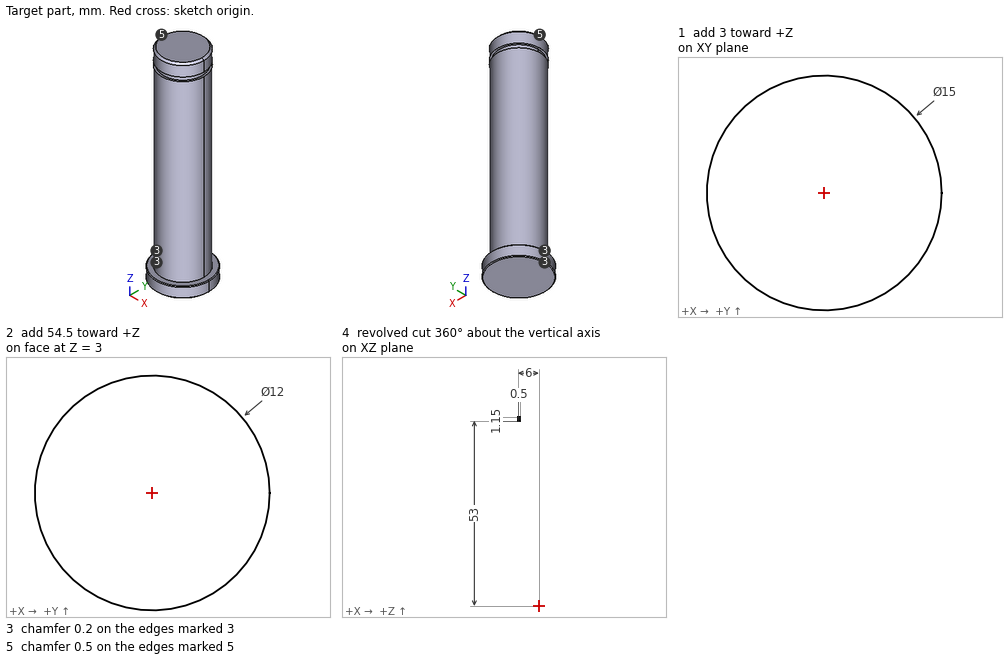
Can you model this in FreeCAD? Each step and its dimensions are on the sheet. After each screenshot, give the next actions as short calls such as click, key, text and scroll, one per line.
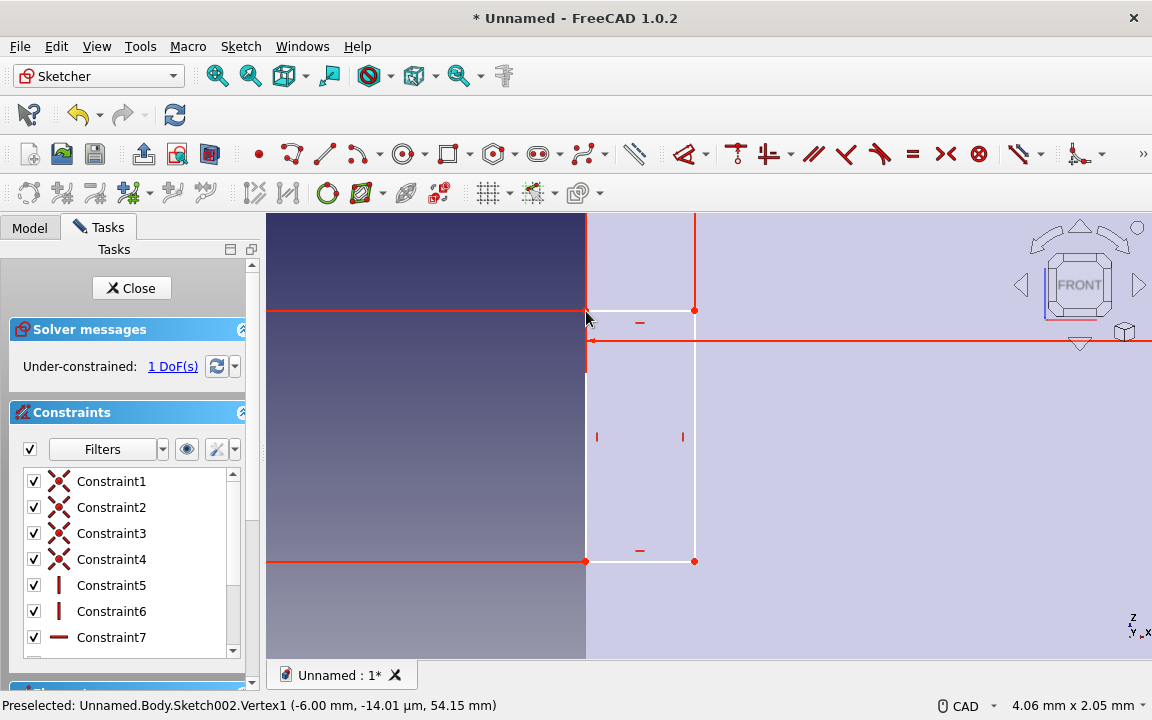
click(586, 562)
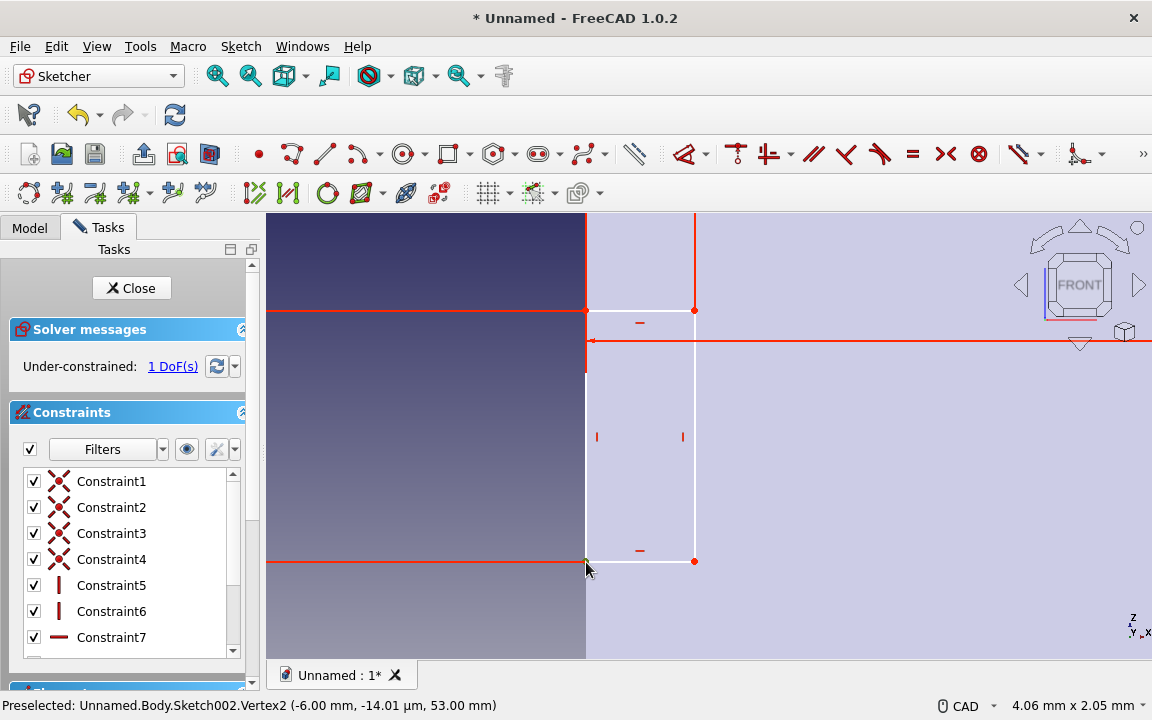
key(i)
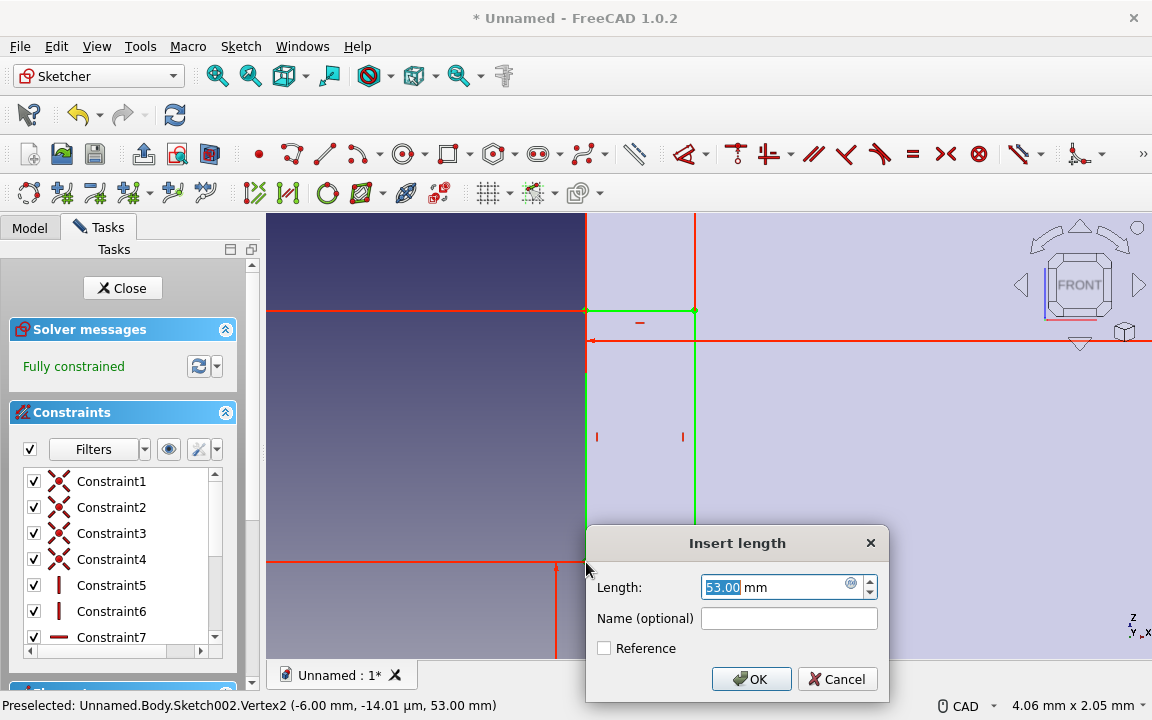
text(53)
key(Return)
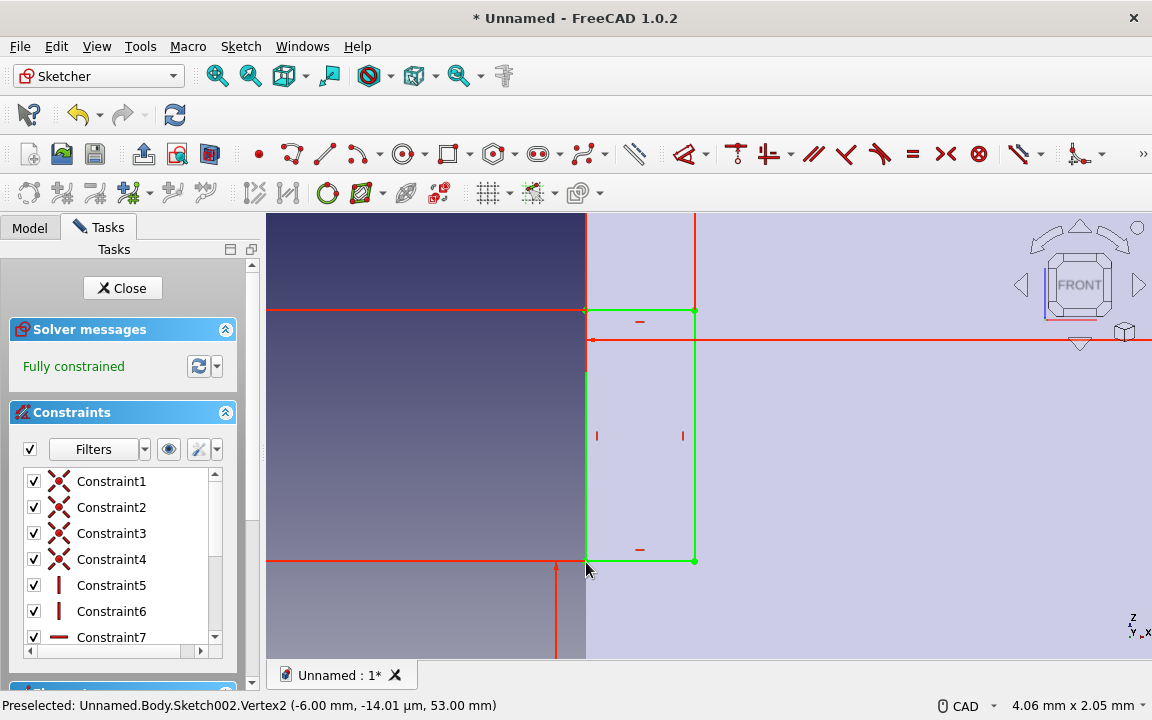
click(123, 288)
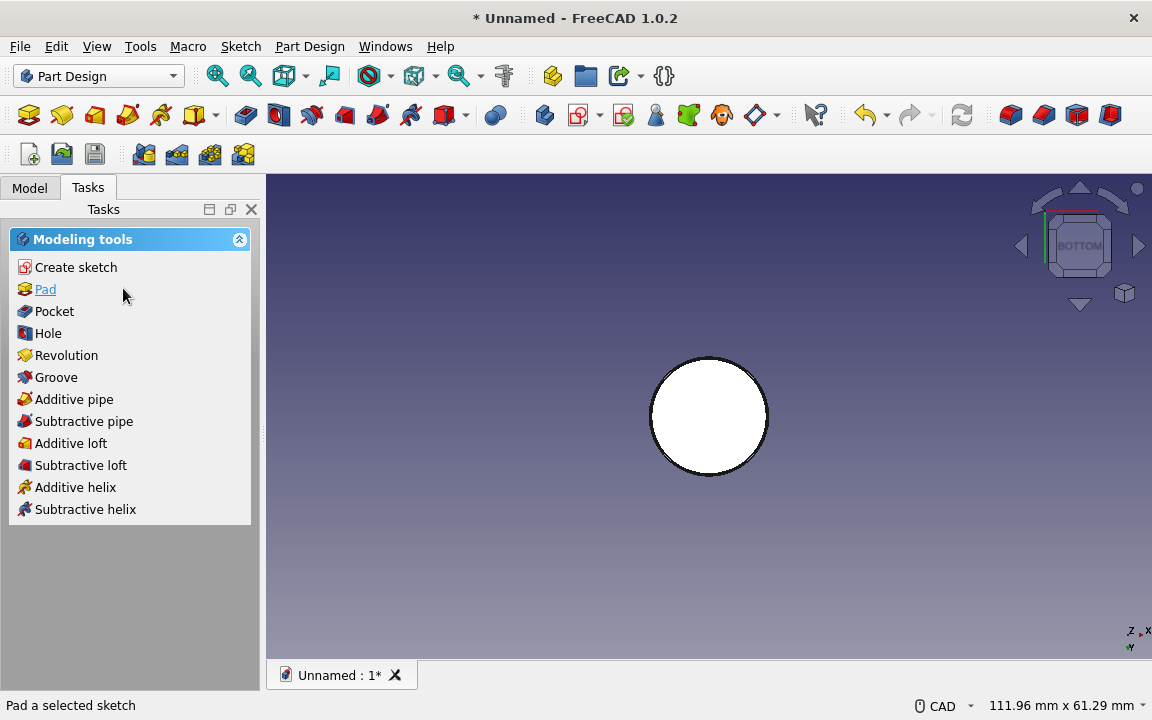
click(312, 116)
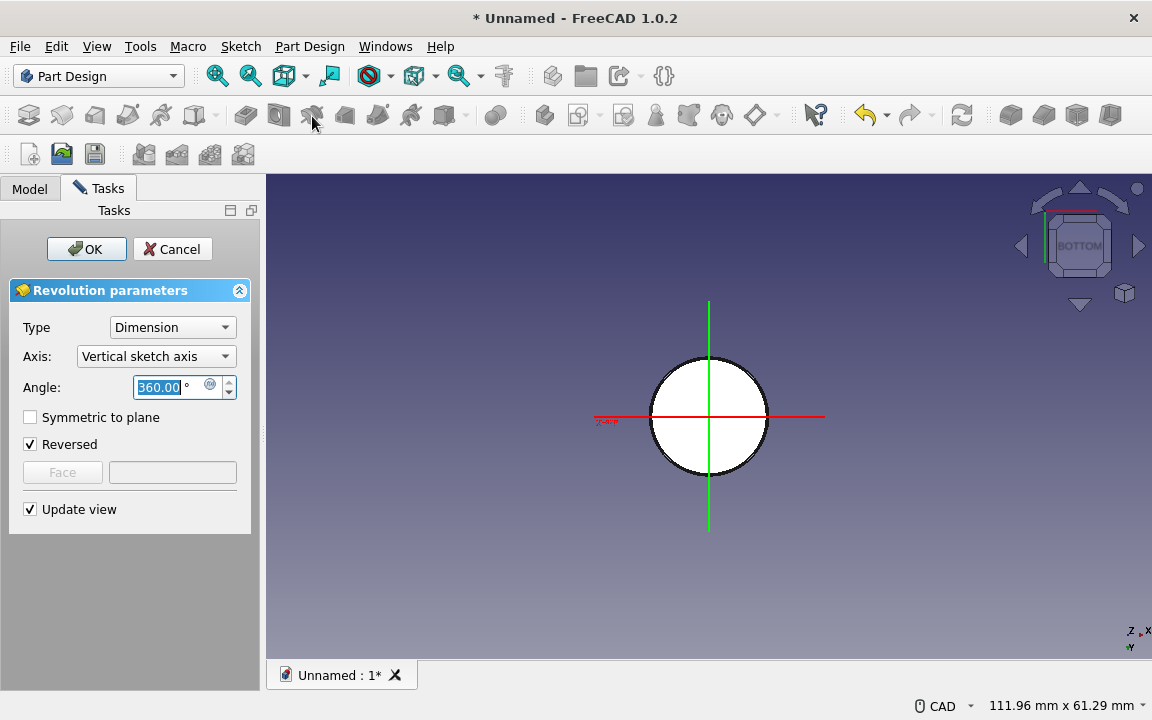
click(87, 249)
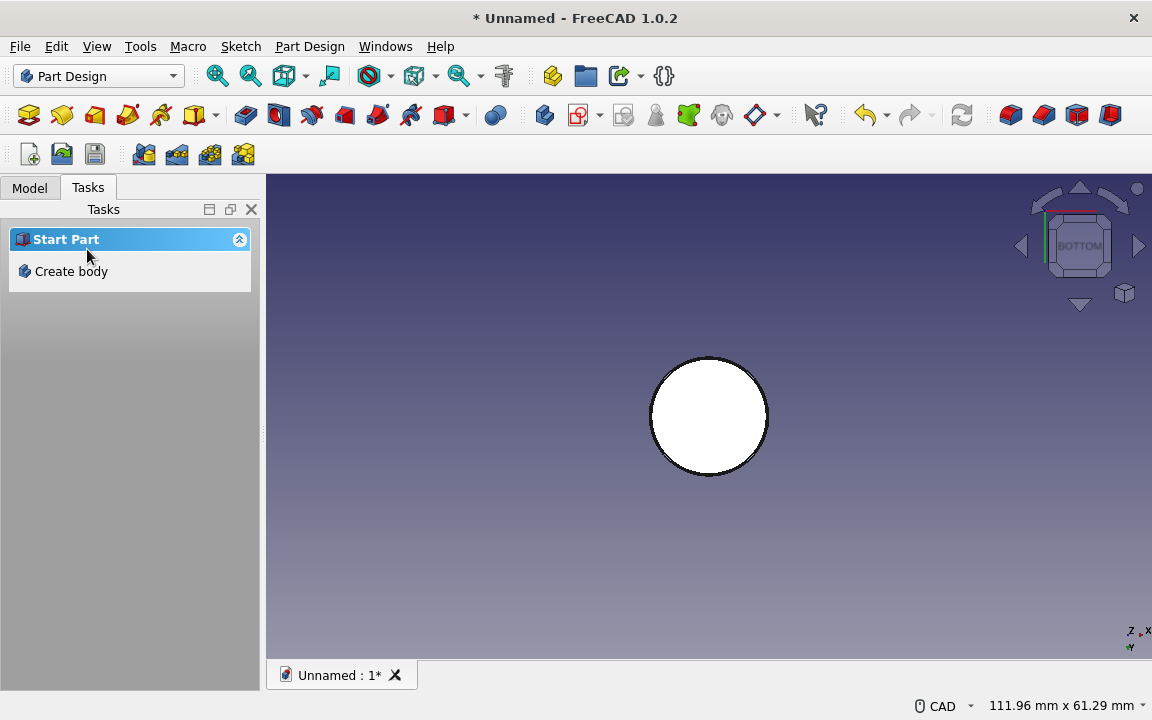
key(v)
key(f)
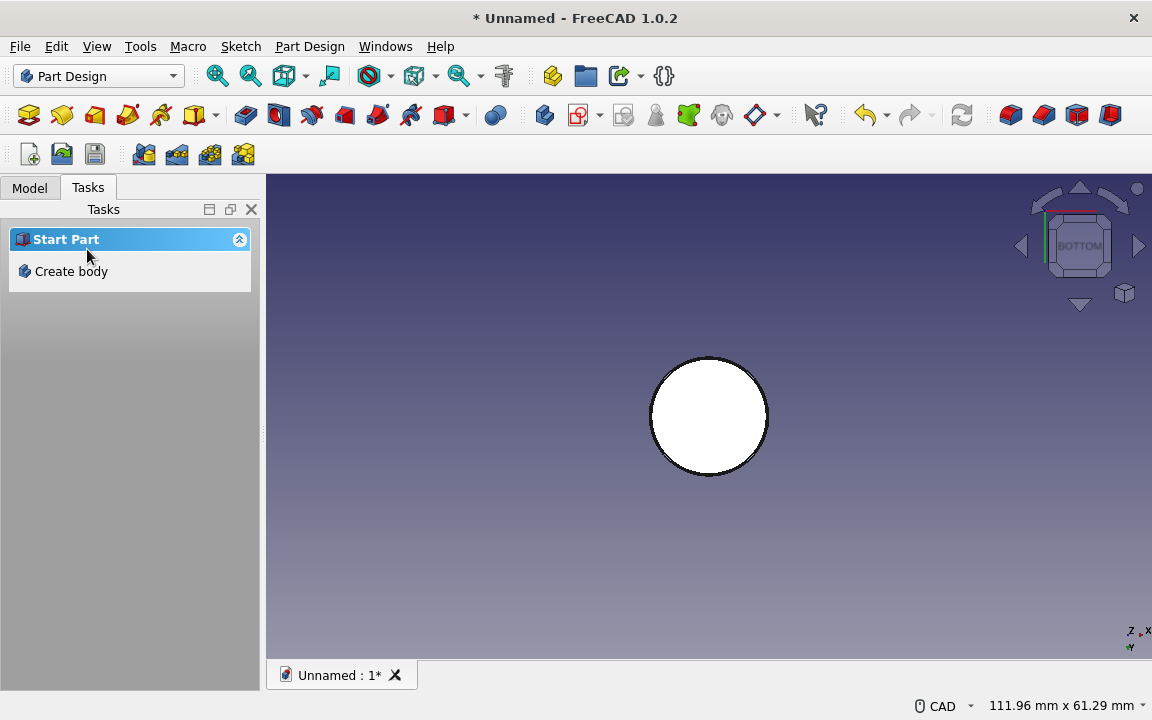
key(0)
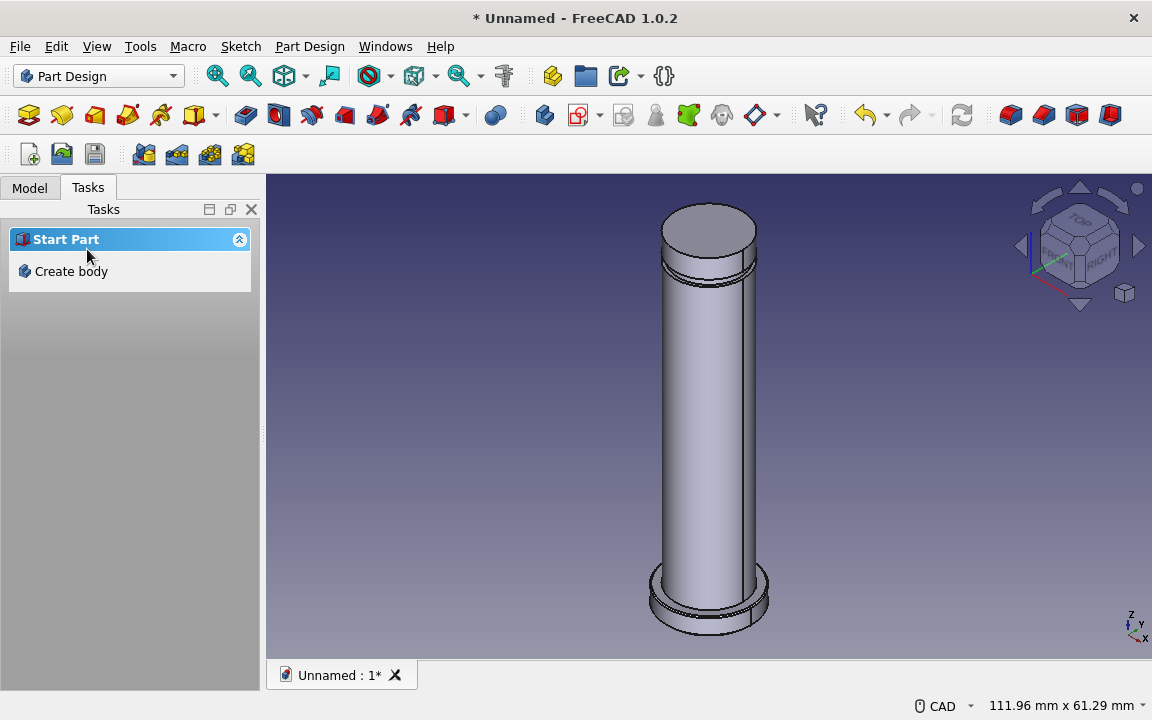
click(667, 242)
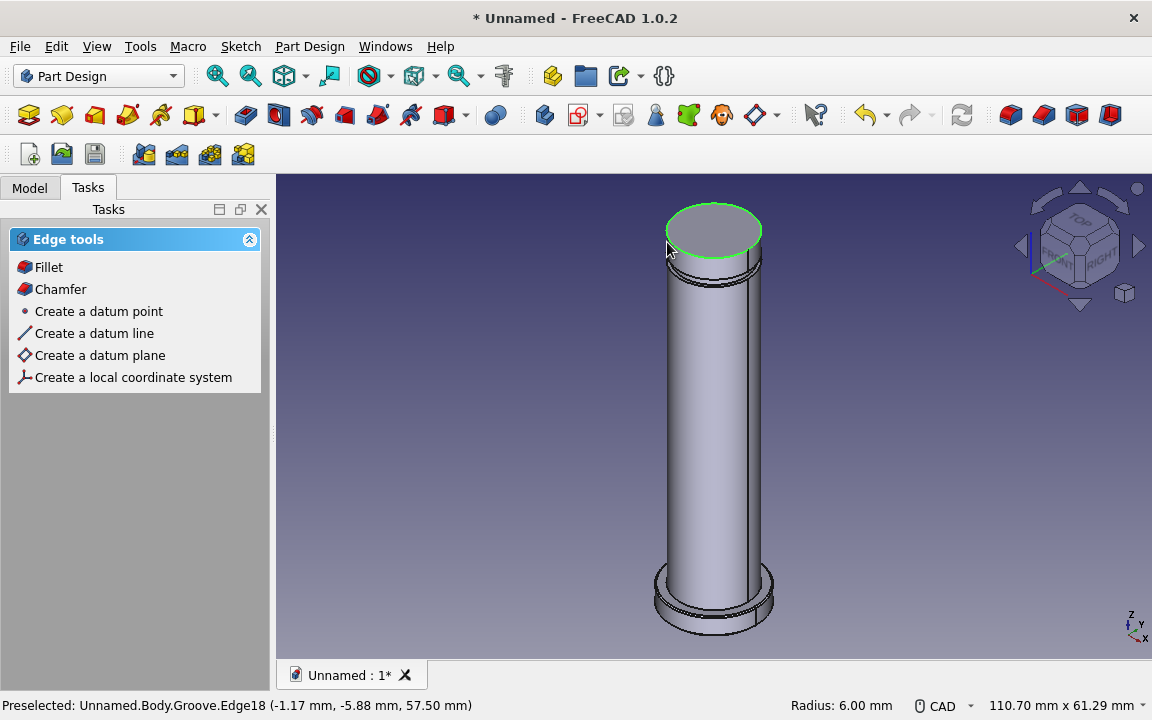
click(1044, 116)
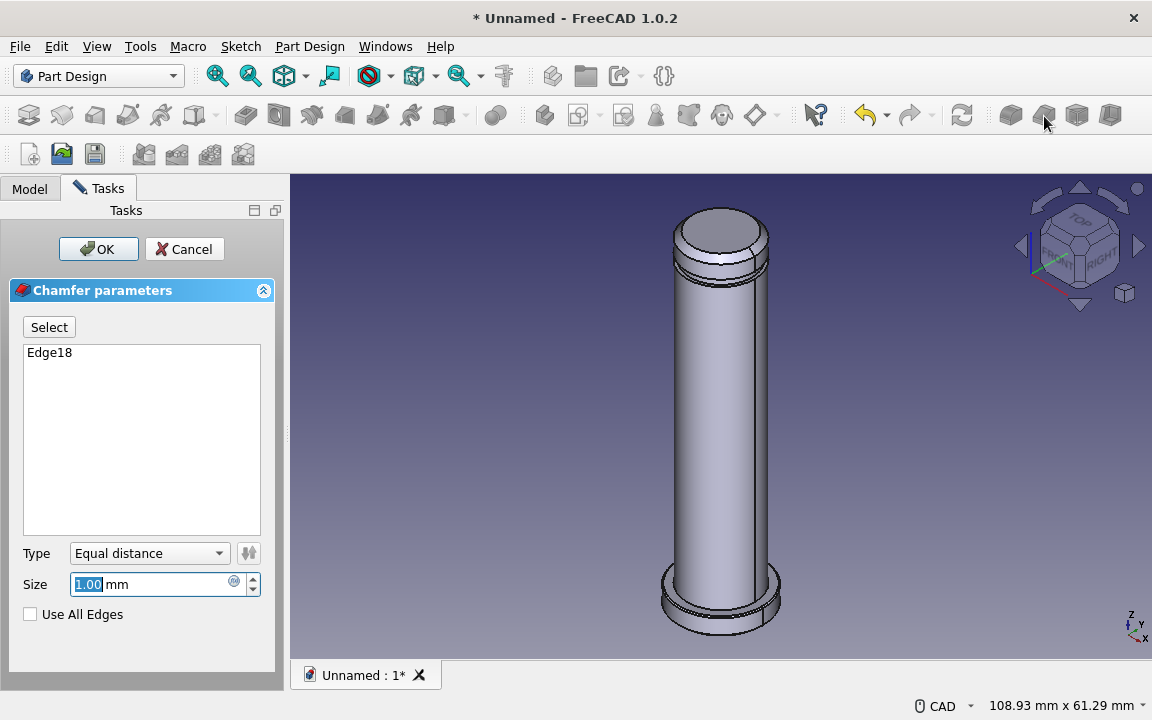
text(0.5)
key(Tab)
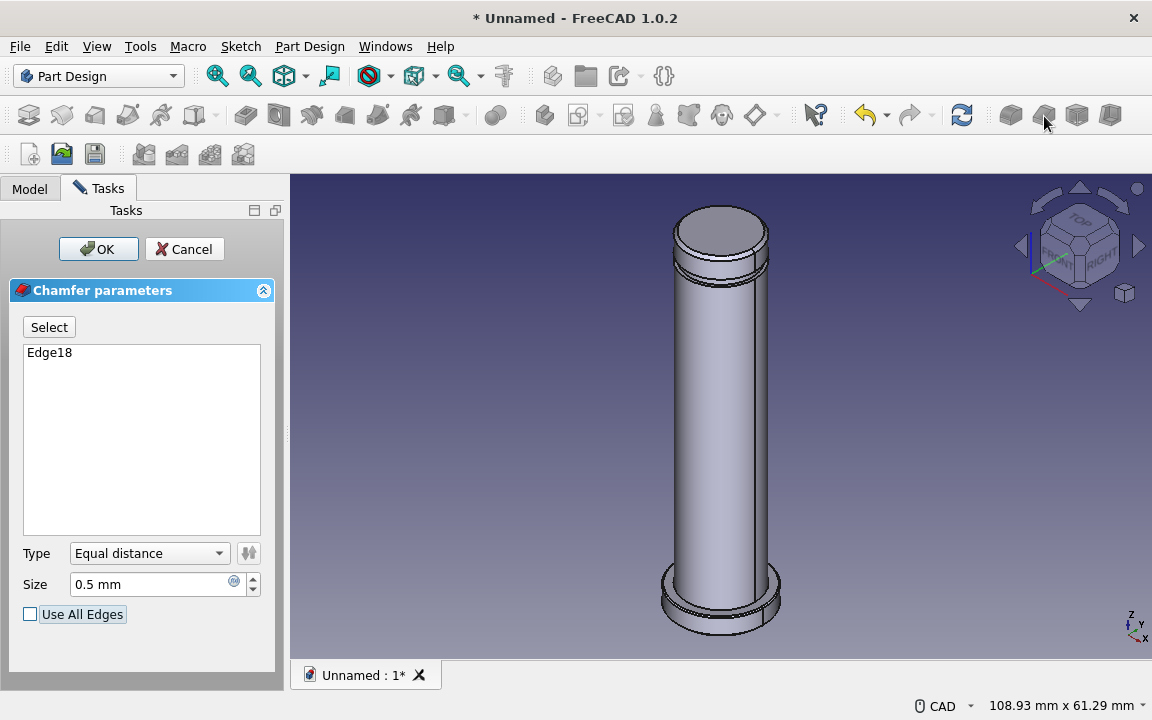
click(99, 249)